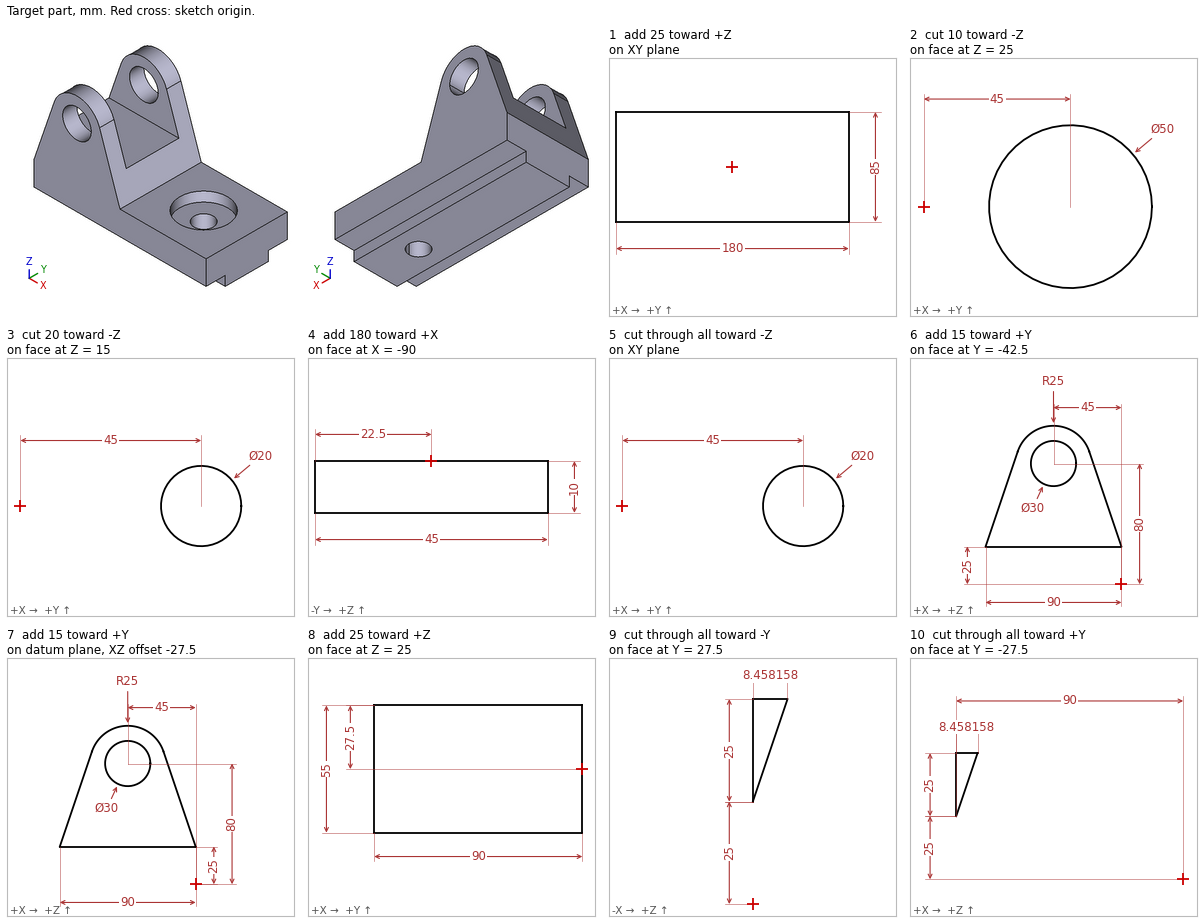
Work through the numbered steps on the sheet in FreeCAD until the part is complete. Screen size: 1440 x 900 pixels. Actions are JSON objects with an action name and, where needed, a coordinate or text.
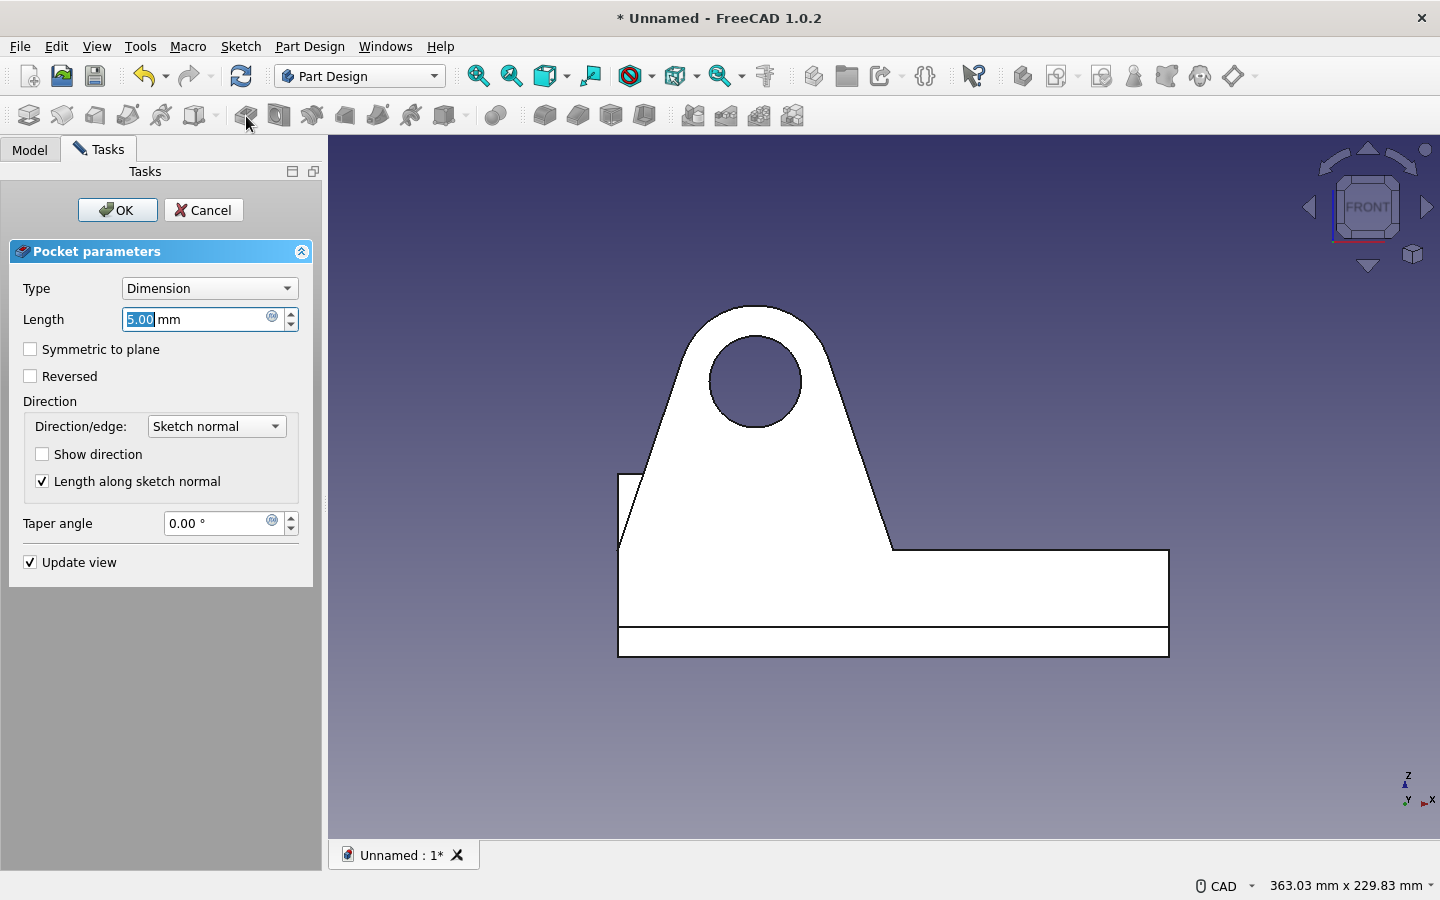
{"action": "left_click", "coordinate": [210, 288]}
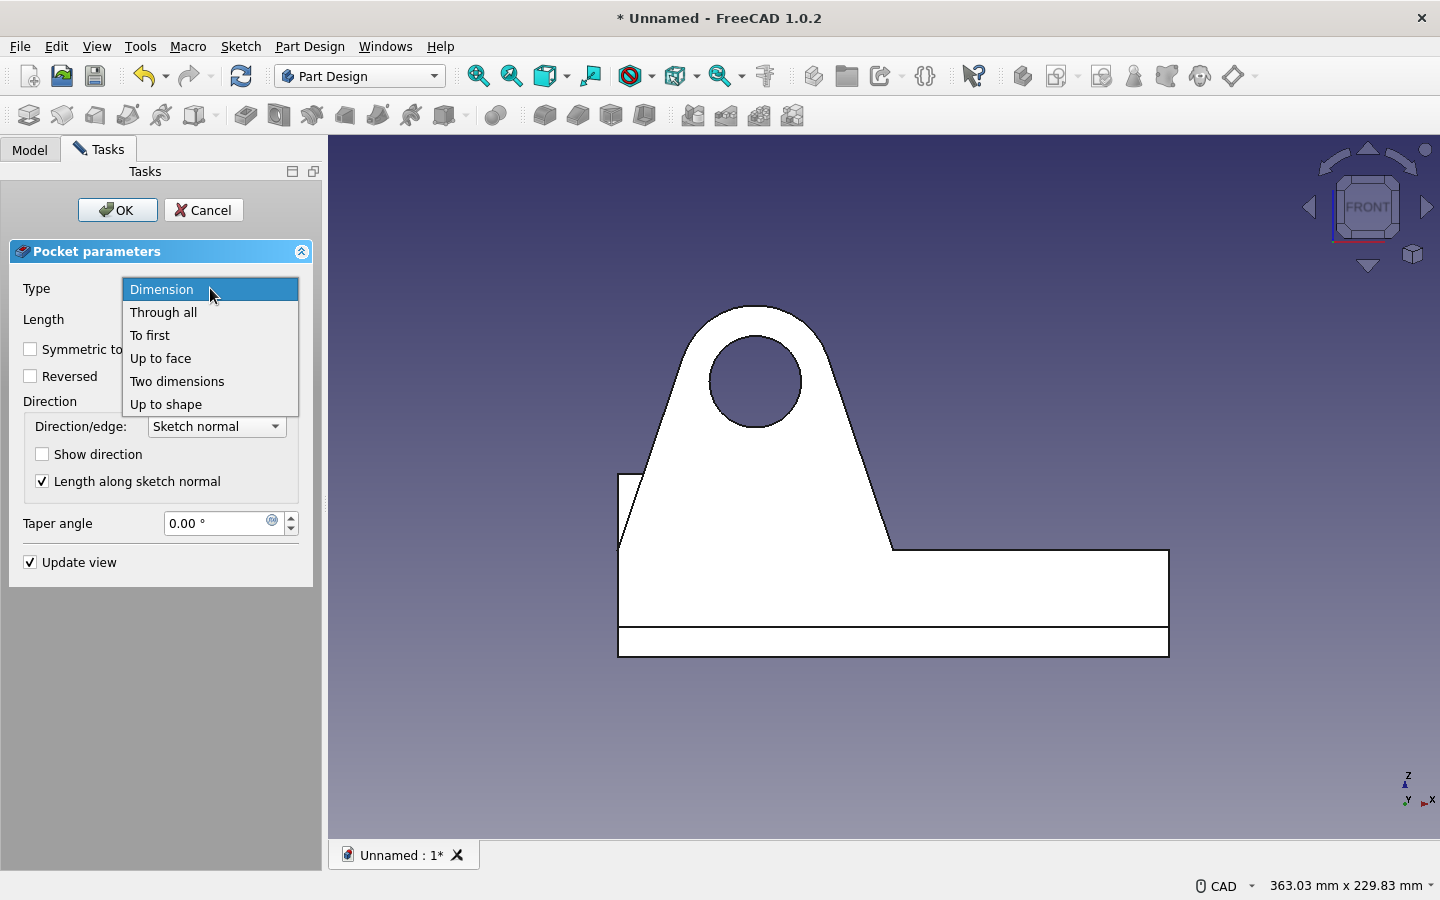
{"action": "left_click", "coordinate": [208, 312]}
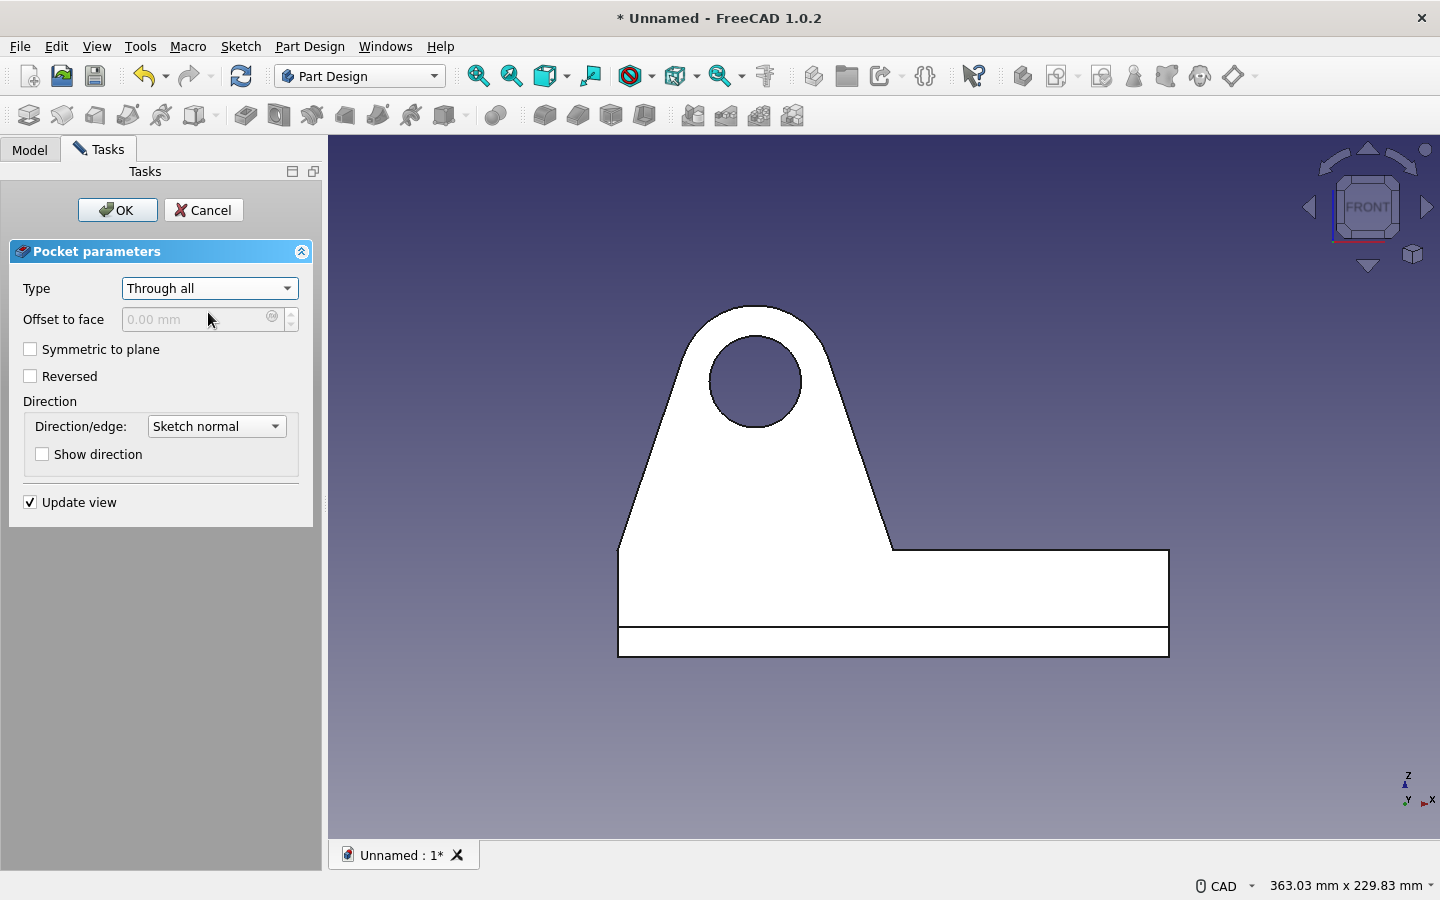
{"action": "left_click", "coordinate": [118, 210]}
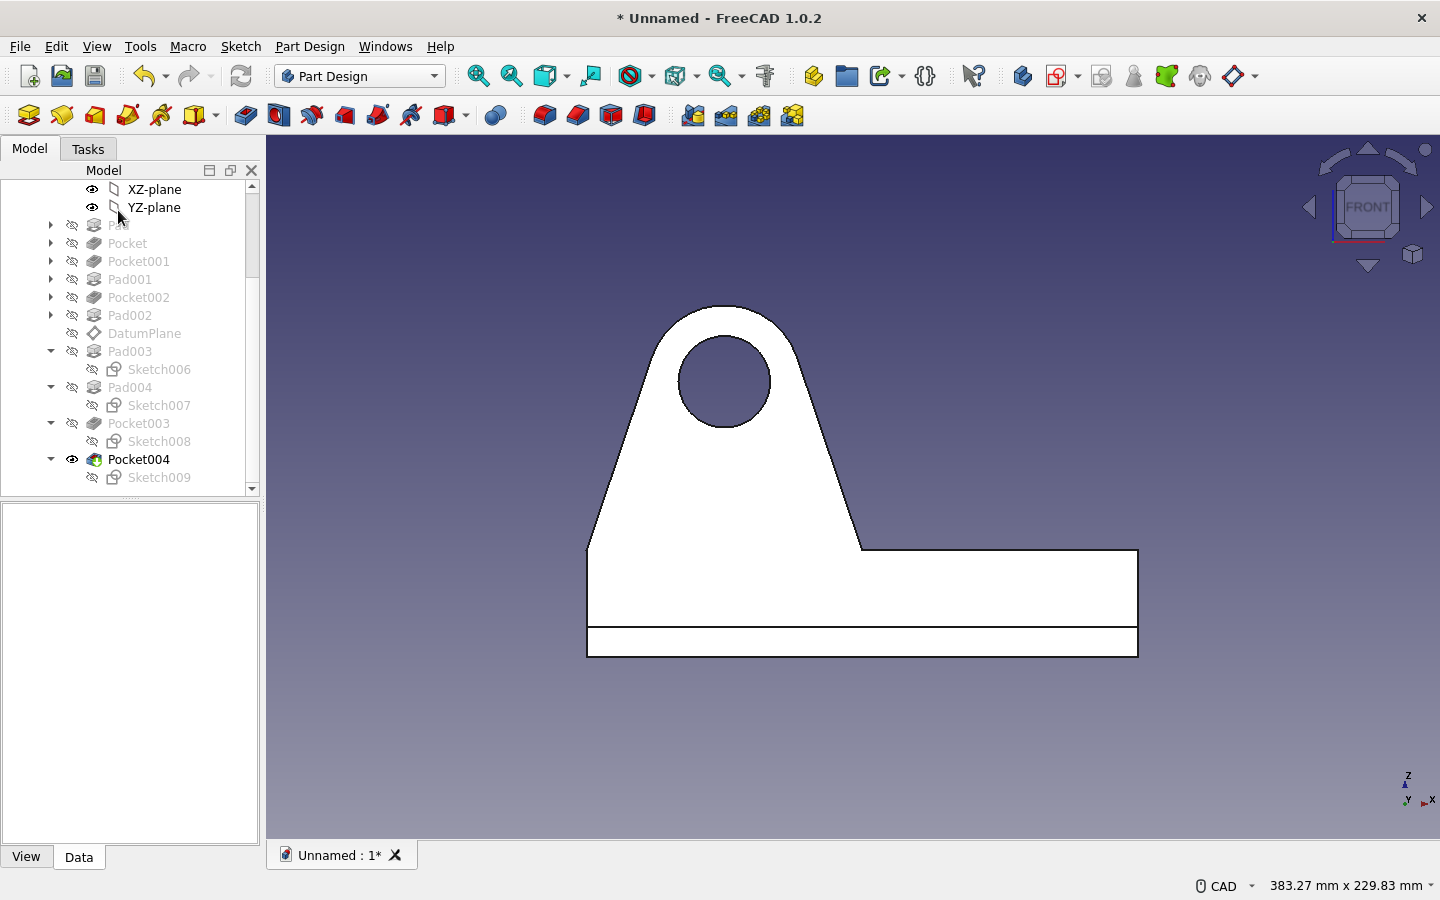
{"action": "key", "text": "0"}